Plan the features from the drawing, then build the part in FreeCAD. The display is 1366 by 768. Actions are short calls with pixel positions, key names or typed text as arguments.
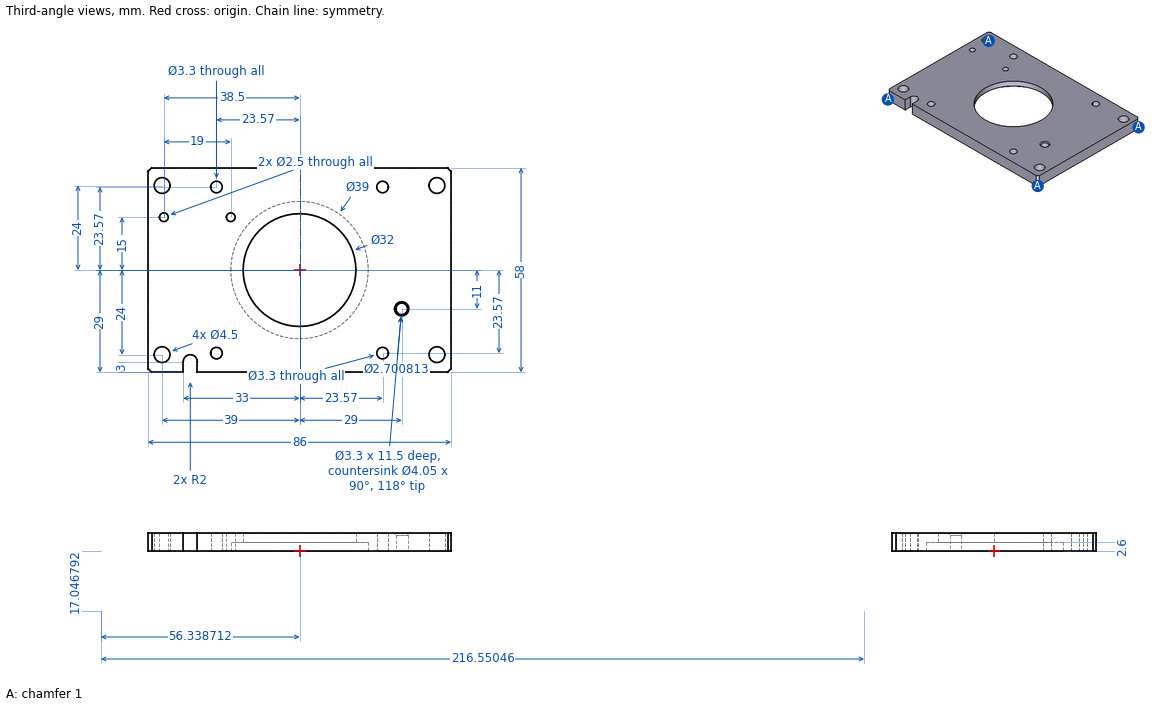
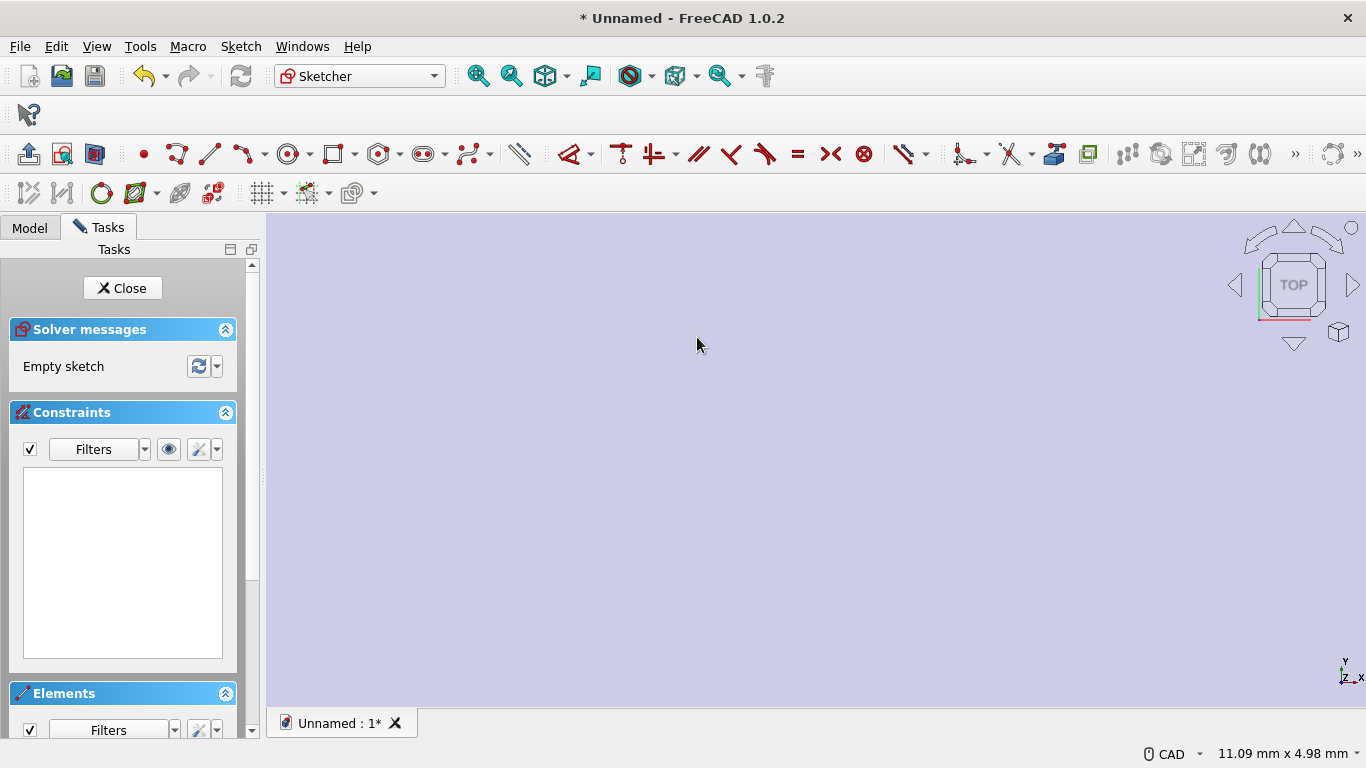
click(288, 154)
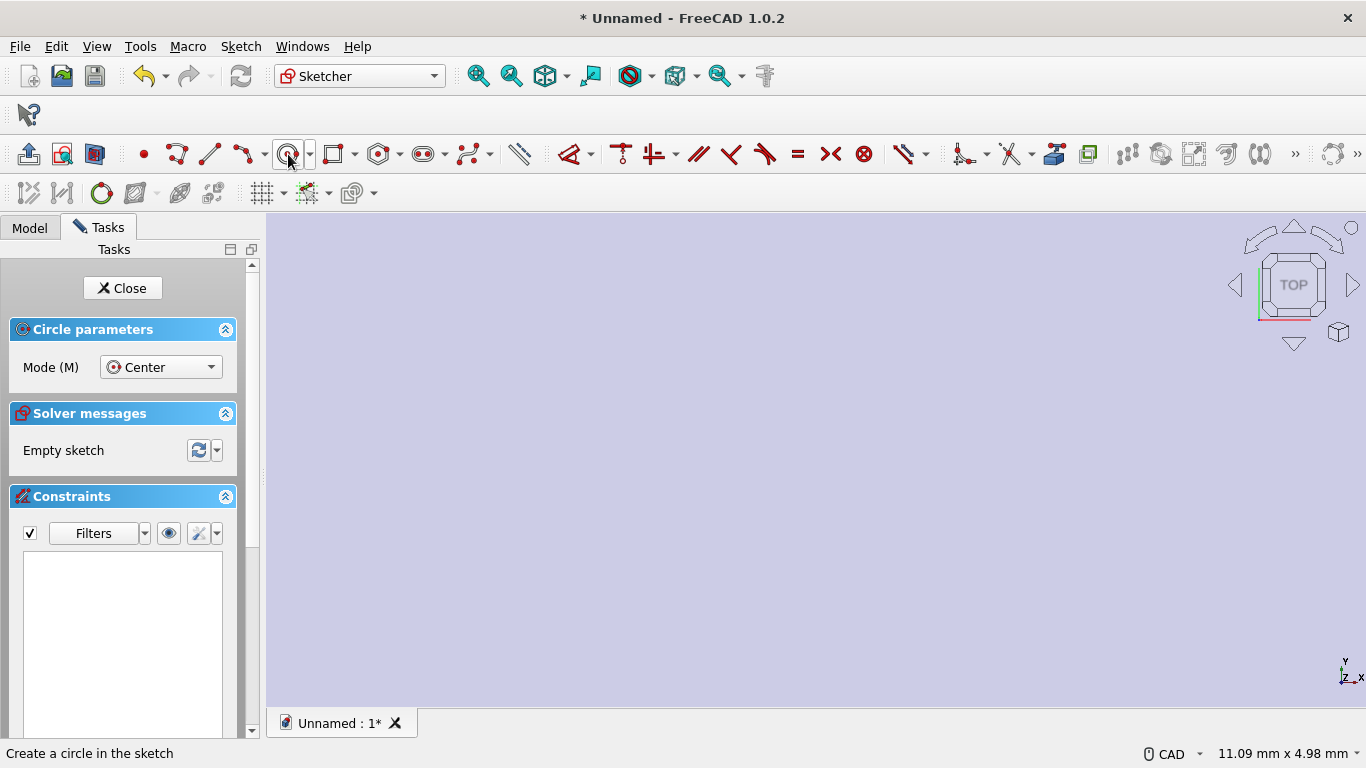
click(741, 464)
move(857, 348)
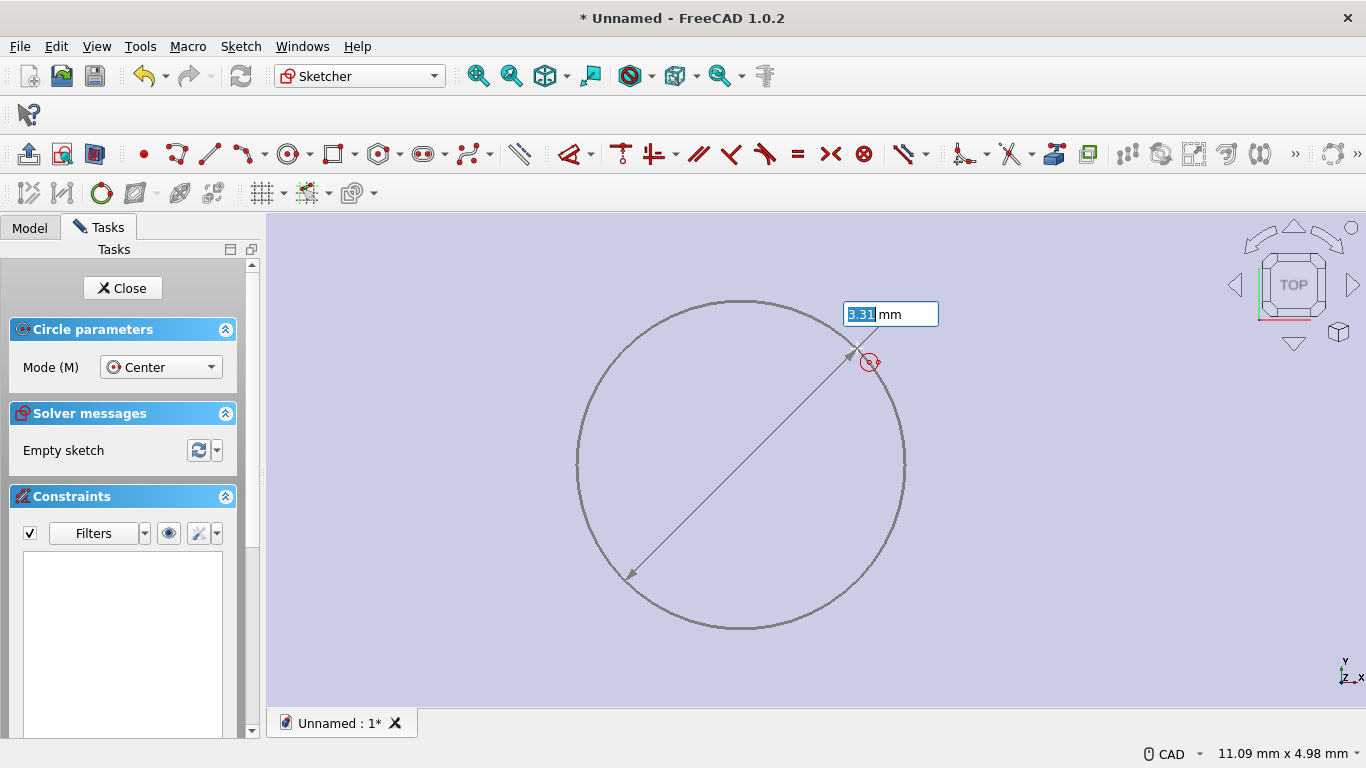
text(3.3)
key(Return)
key(Escape)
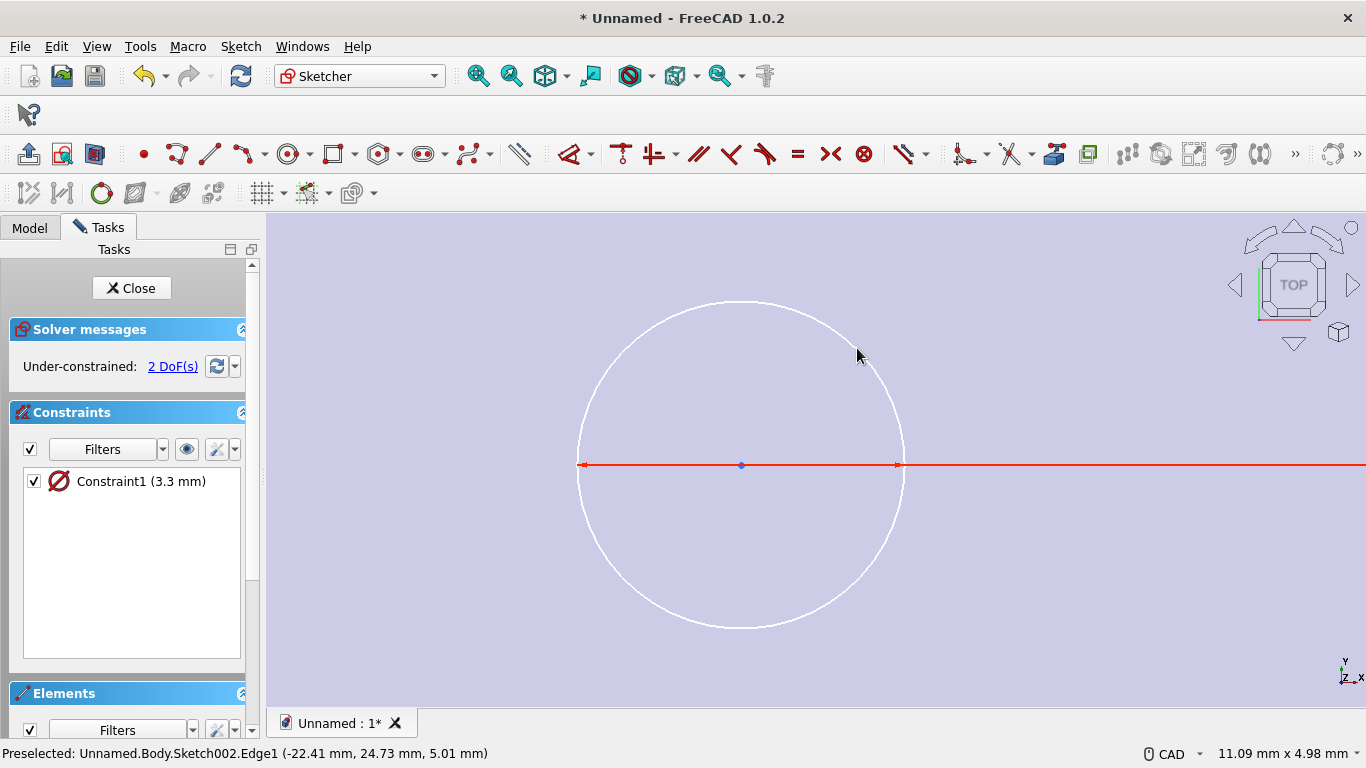
click(568, 154)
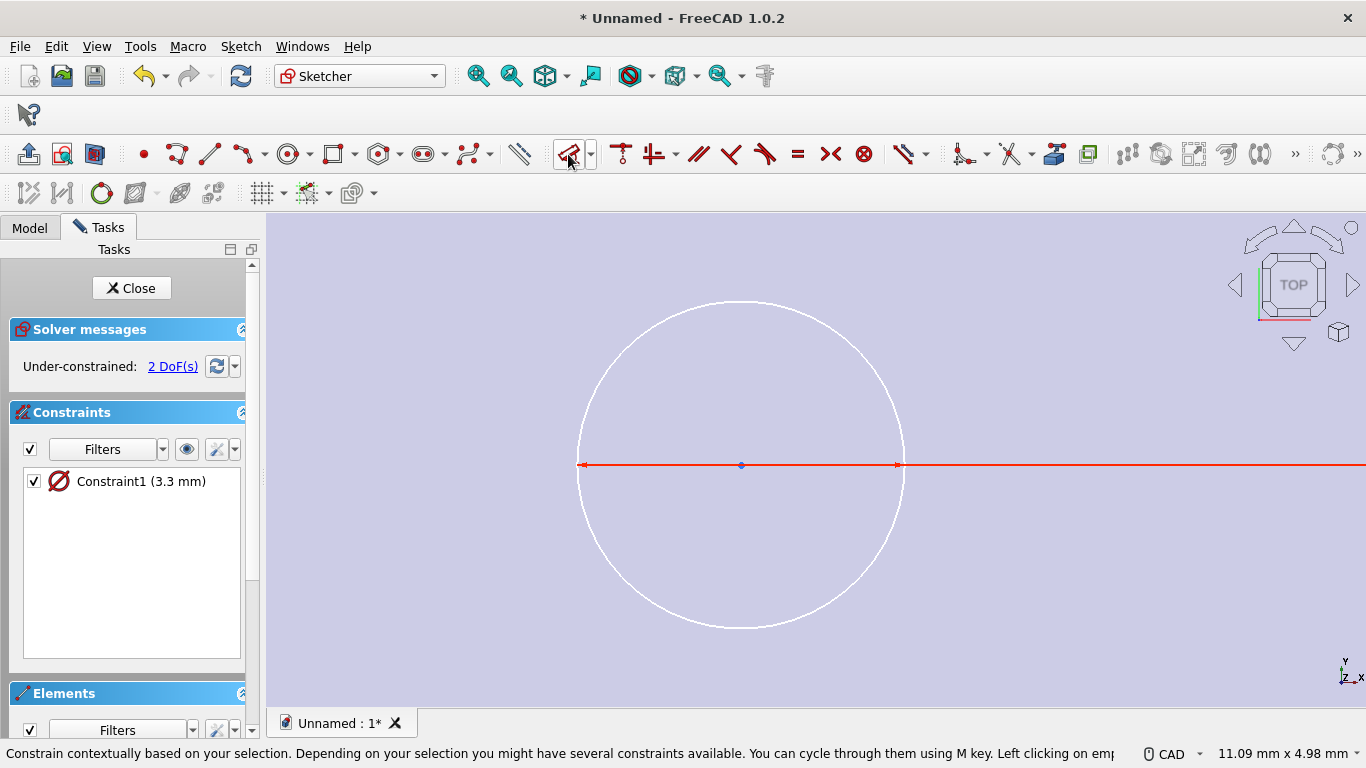
click(741, 465)
click(971, 431)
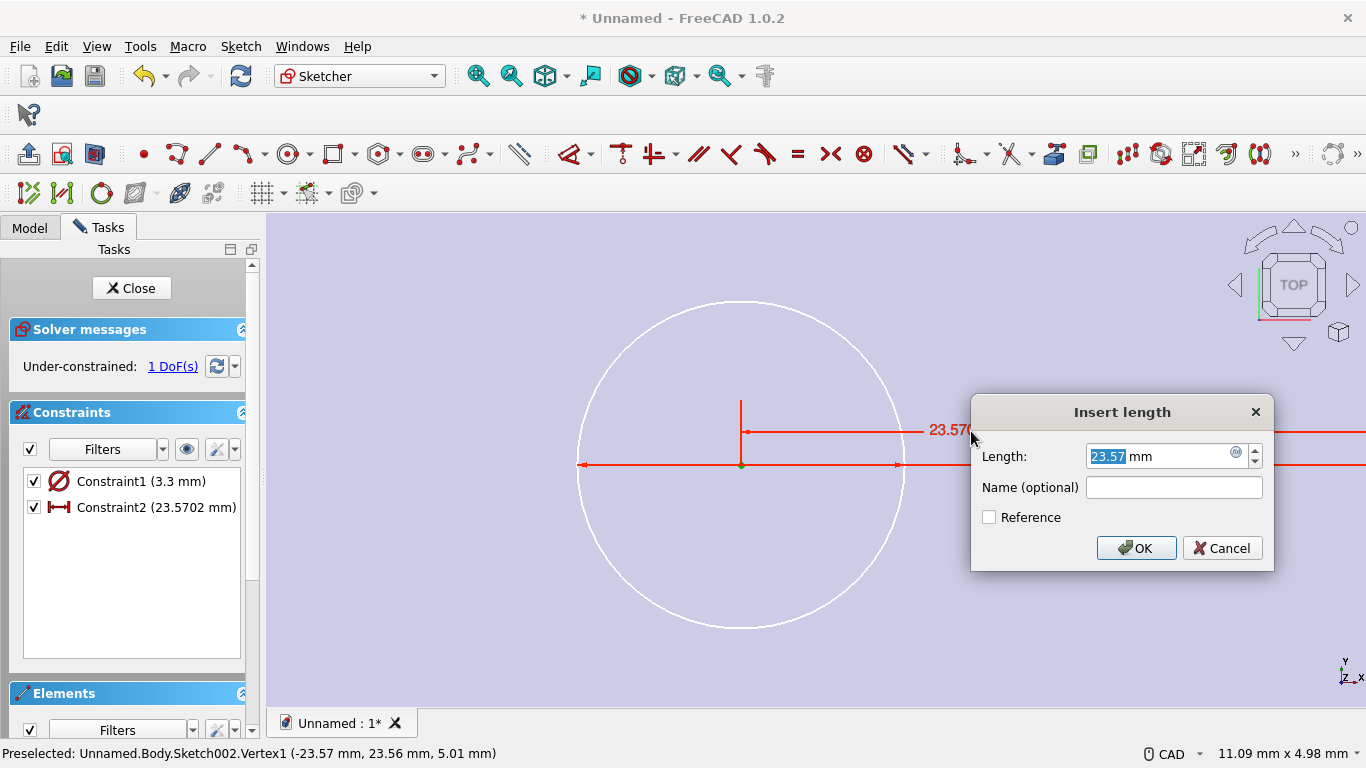
text(23.57)
key(Return)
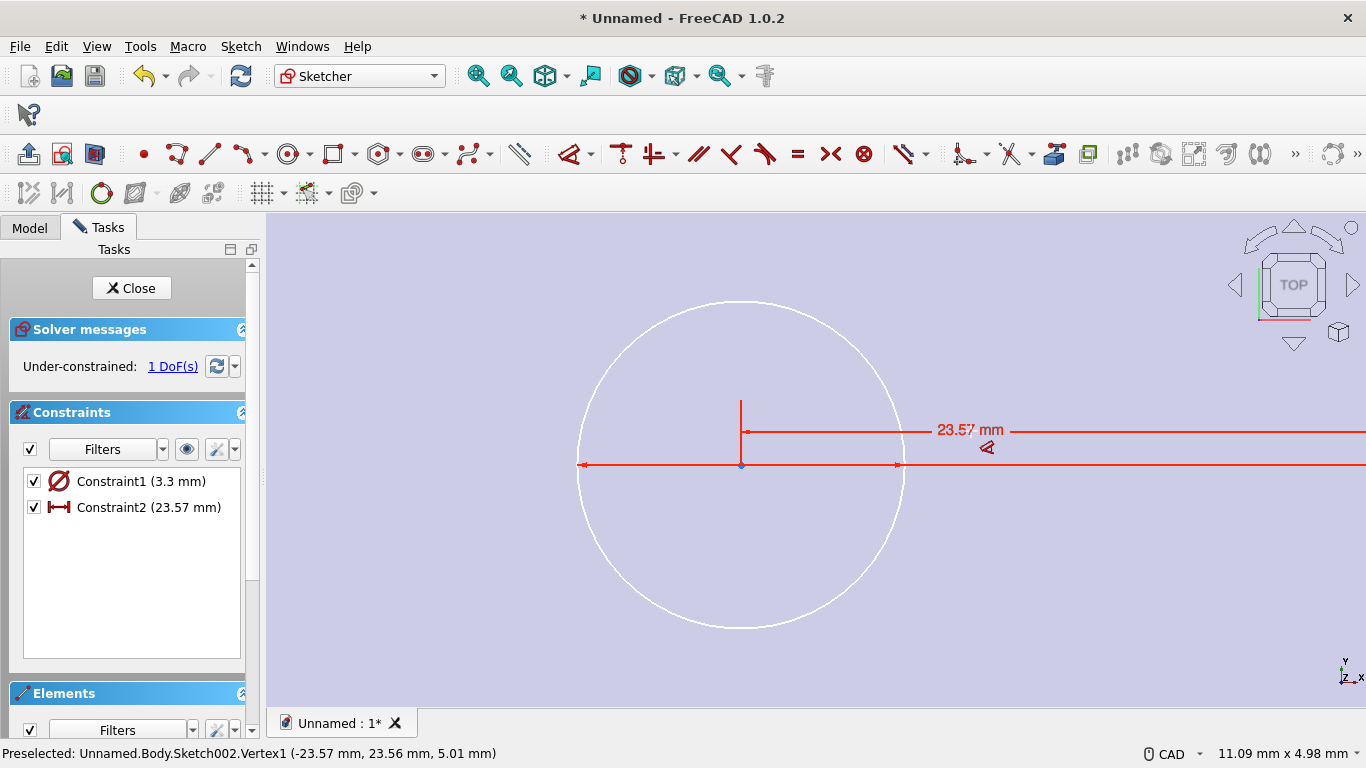
click(741, 465)
click(707, 572)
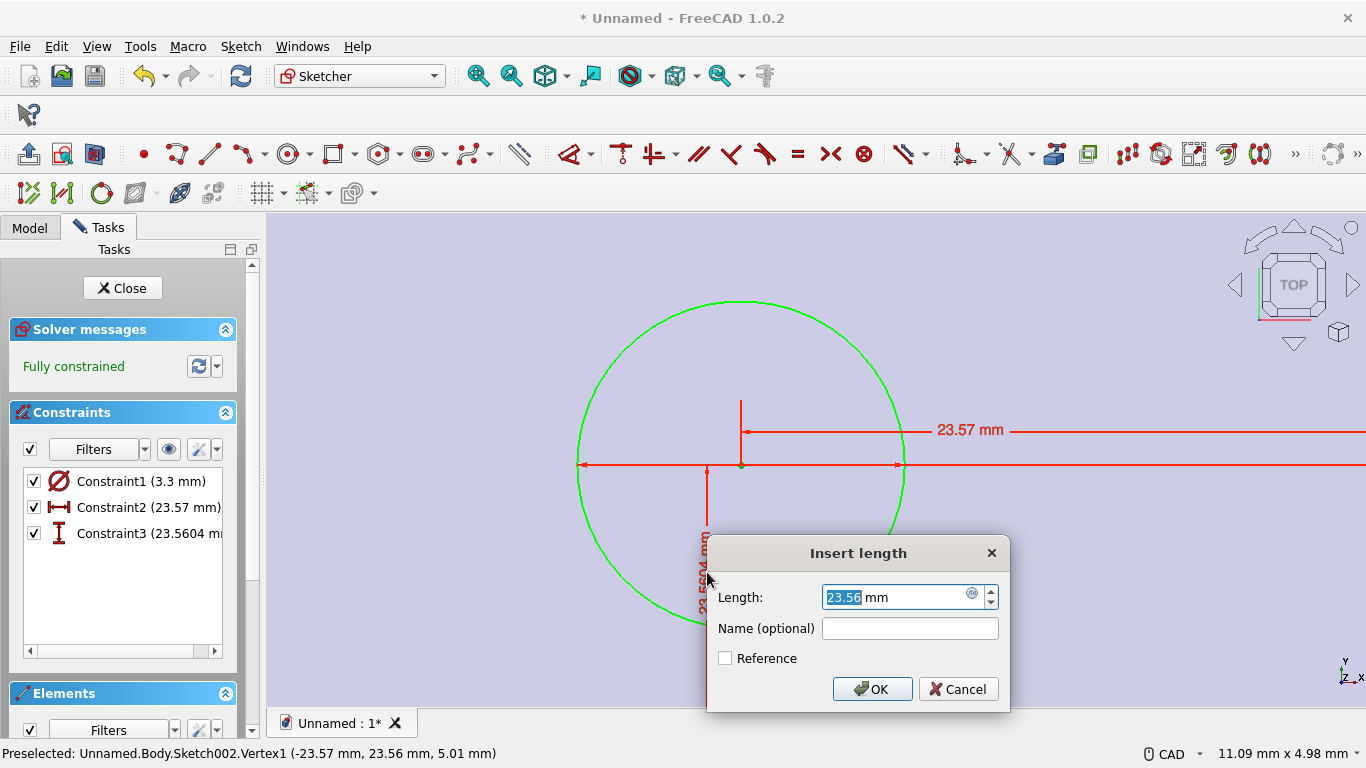
text(23.57)
key(Return)
key(Escape)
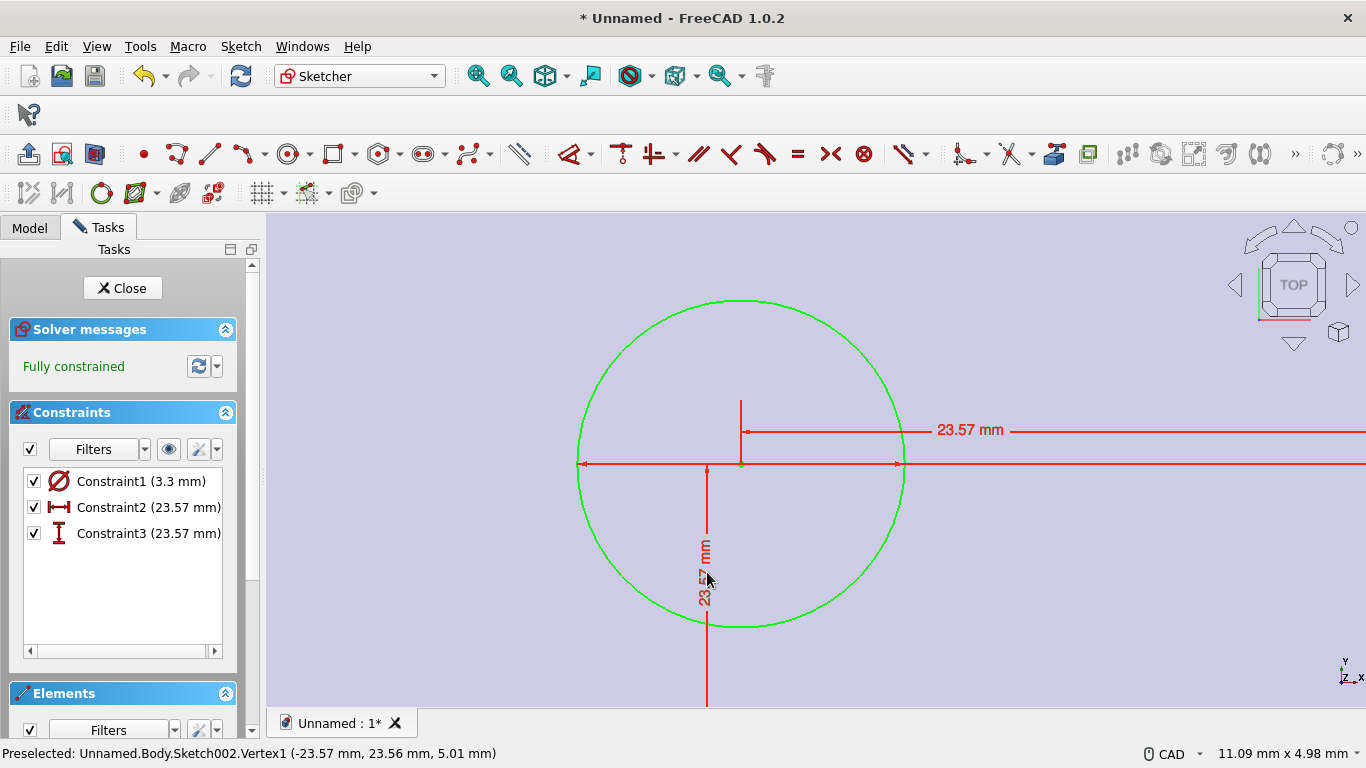
click(123, 288)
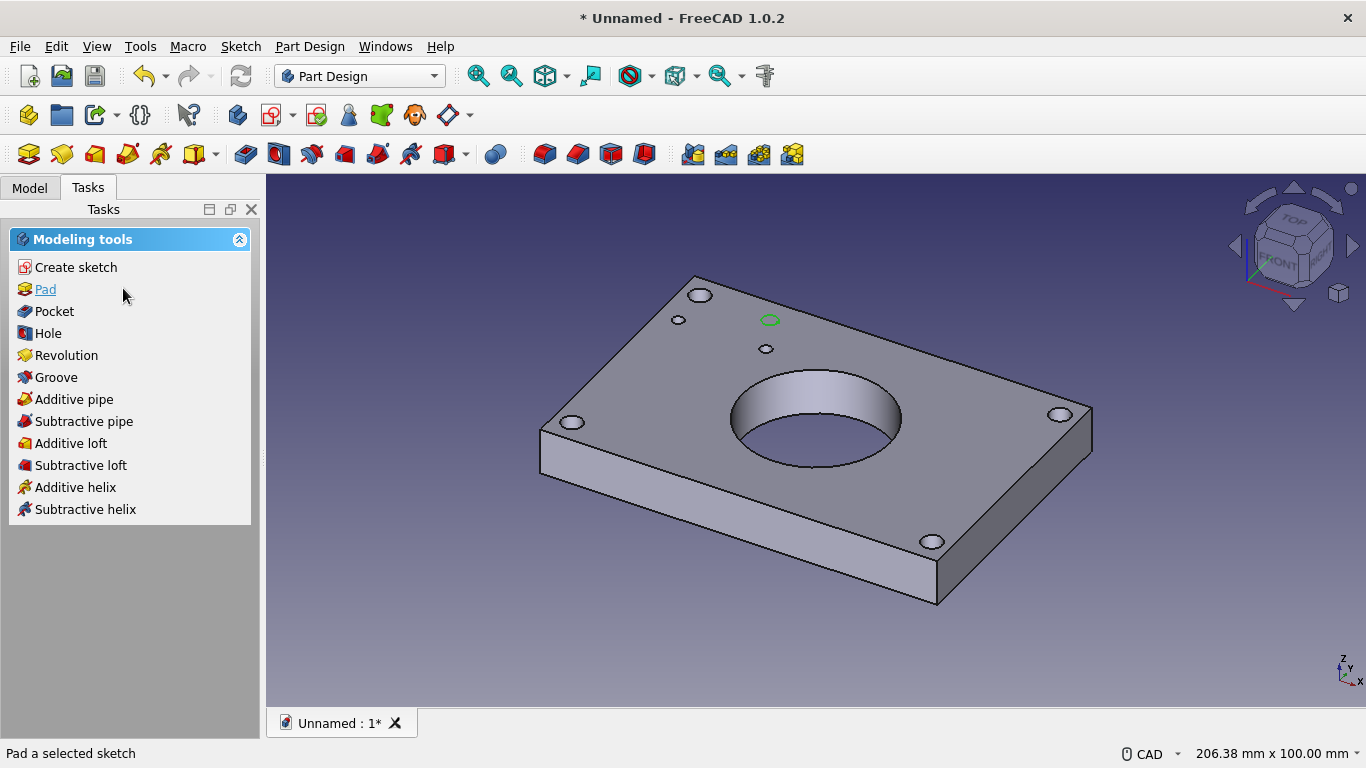
click(279, 154)